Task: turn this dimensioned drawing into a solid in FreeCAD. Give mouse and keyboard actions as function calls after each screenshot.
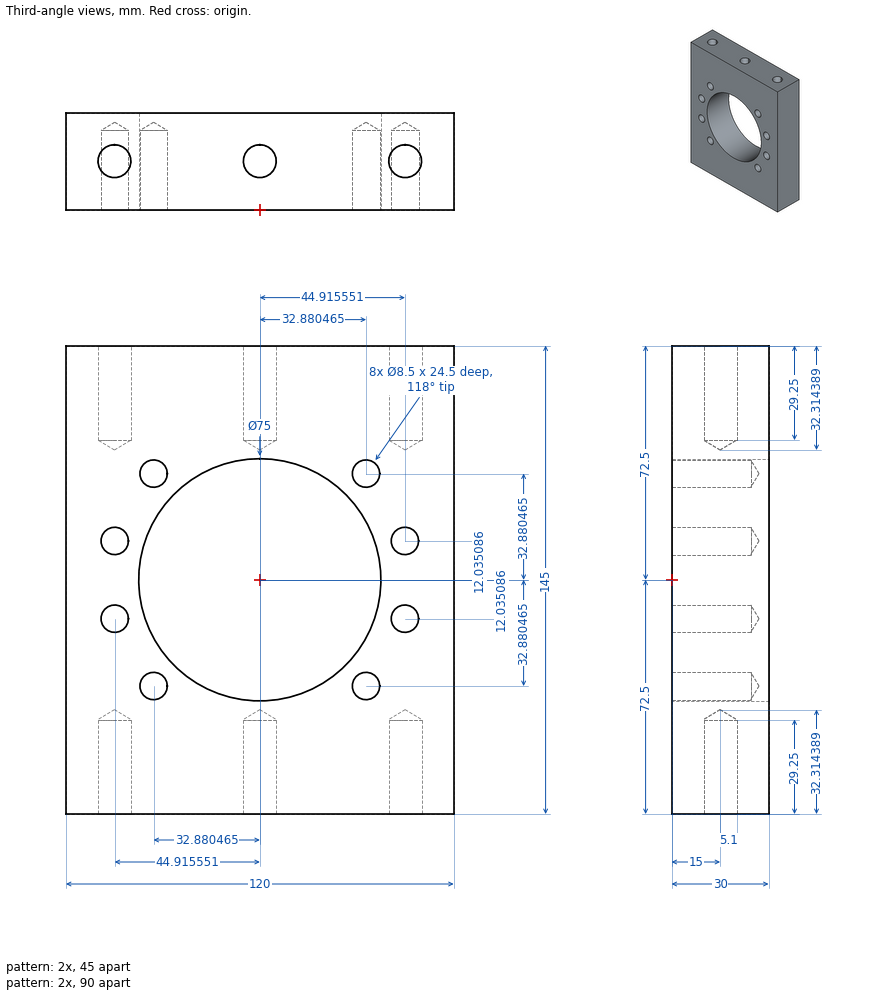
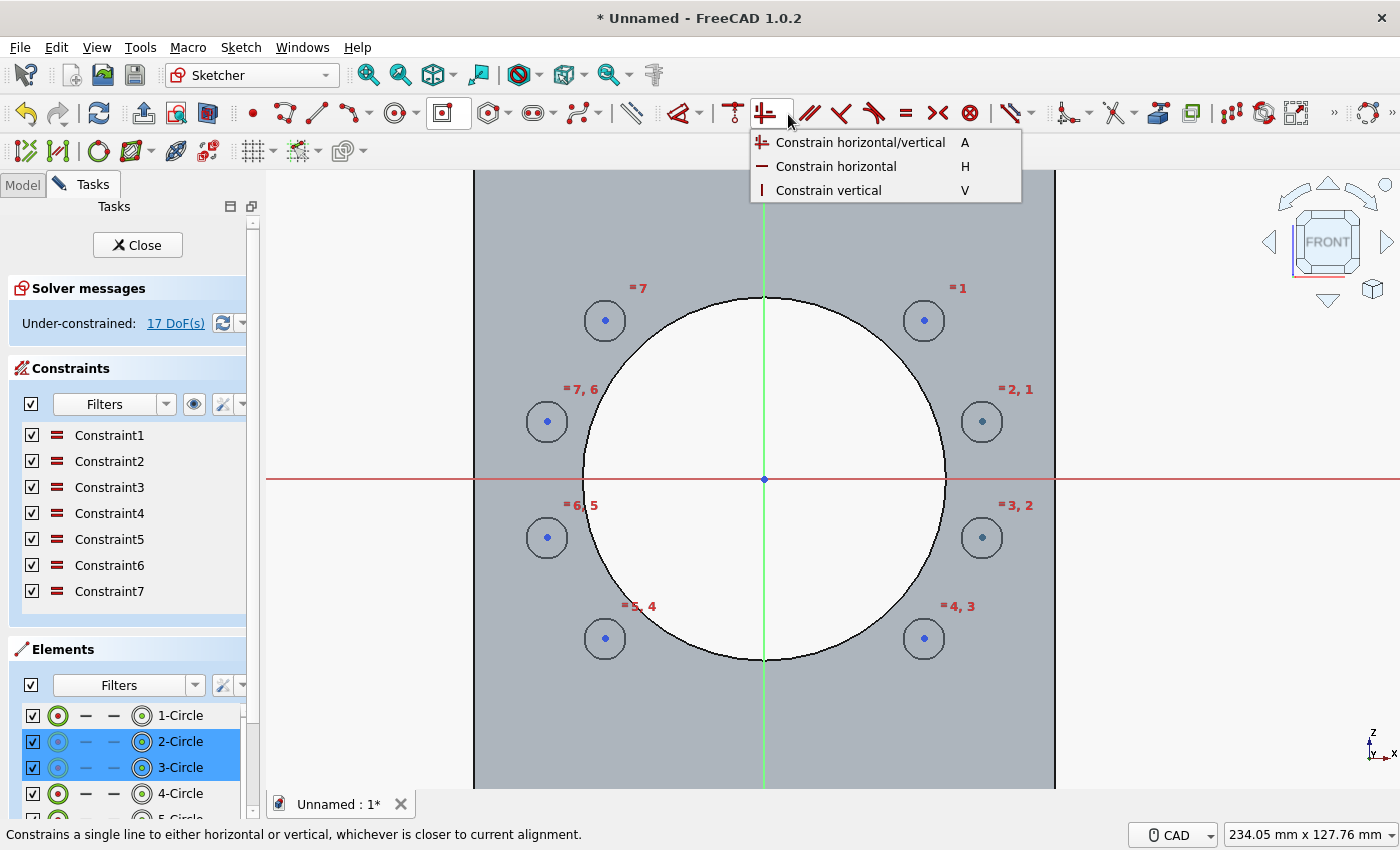
click(886, 190)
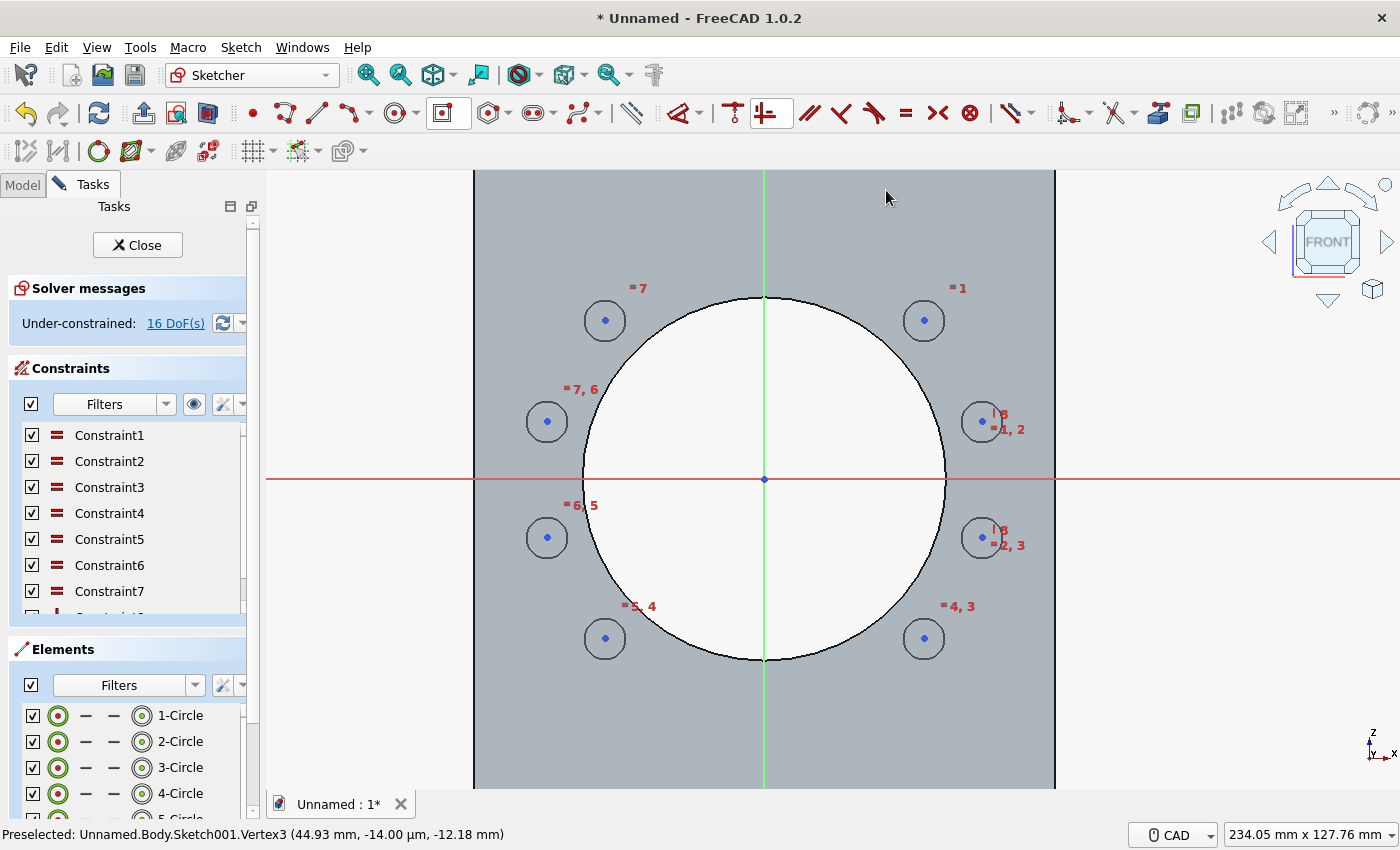
click(924, 321)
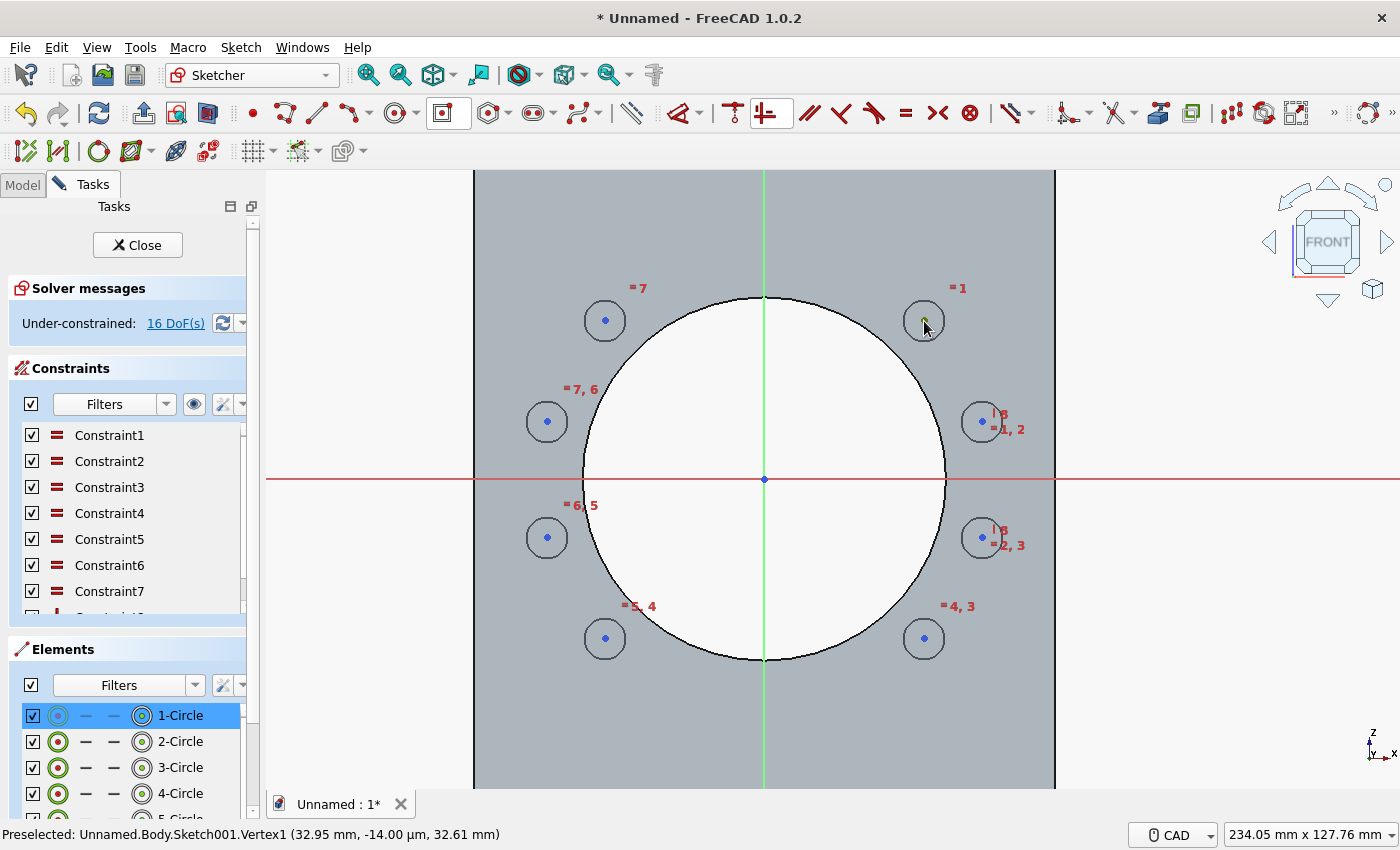
click(924, 639)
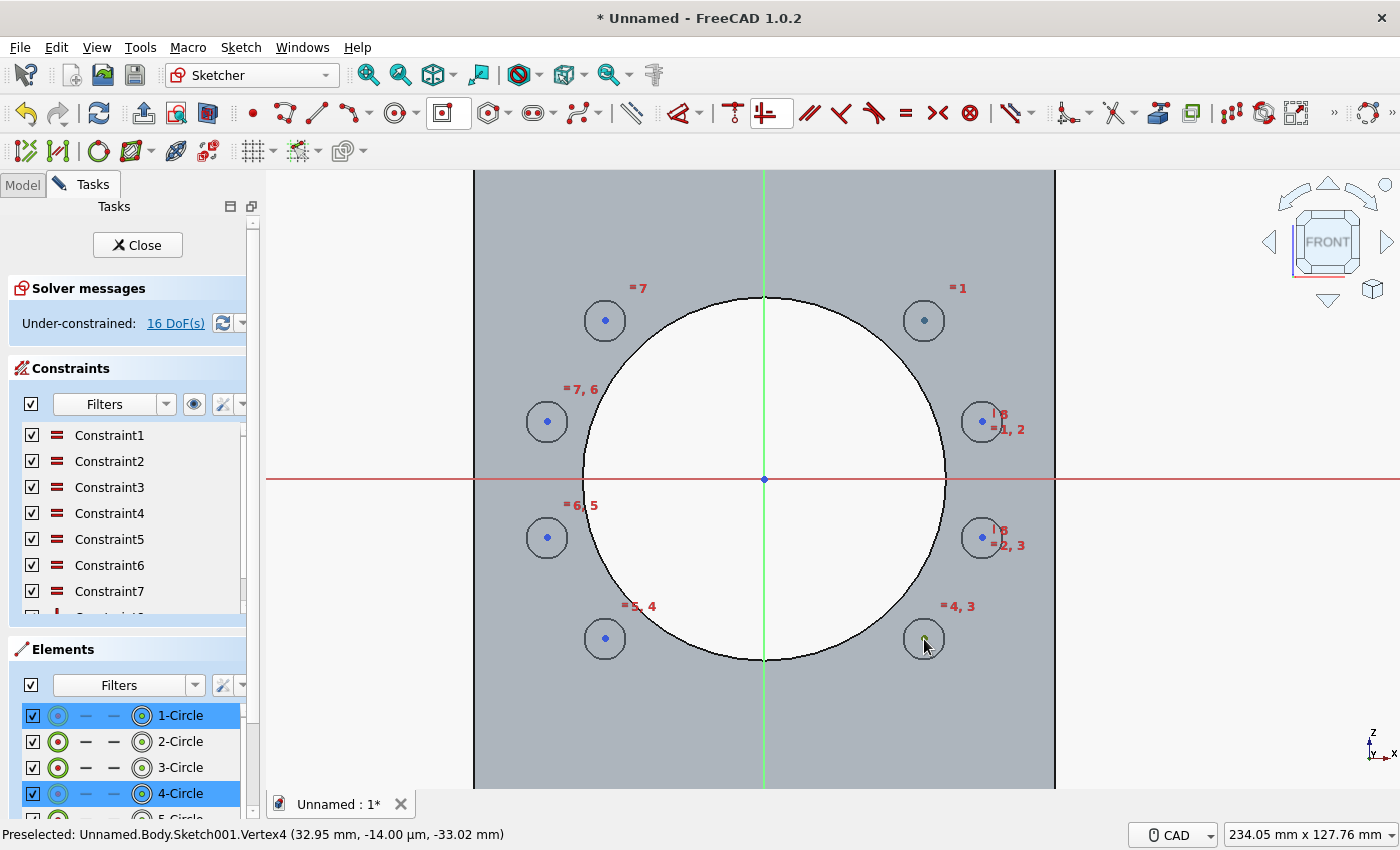
click(788, 114)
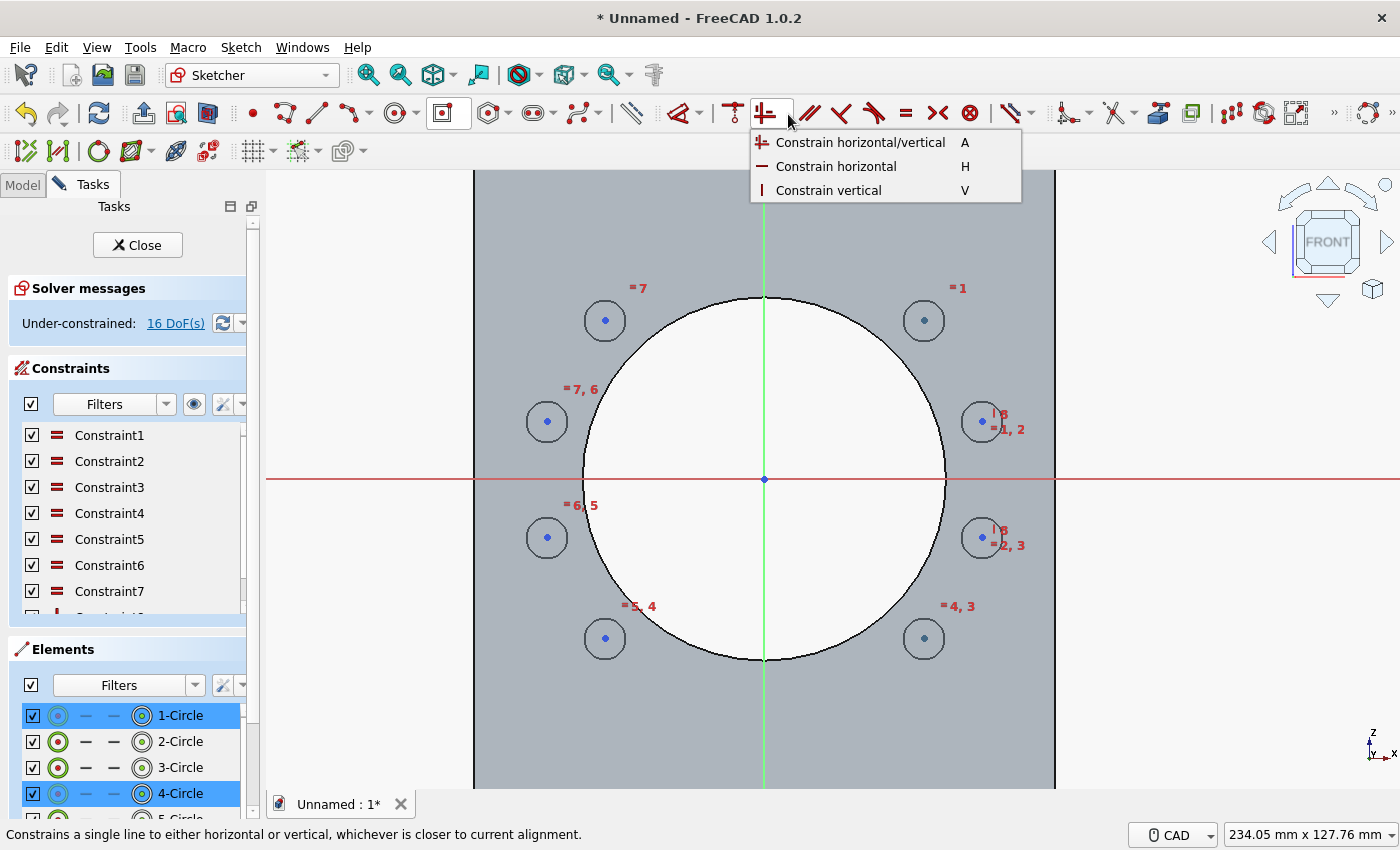
click(886, 190)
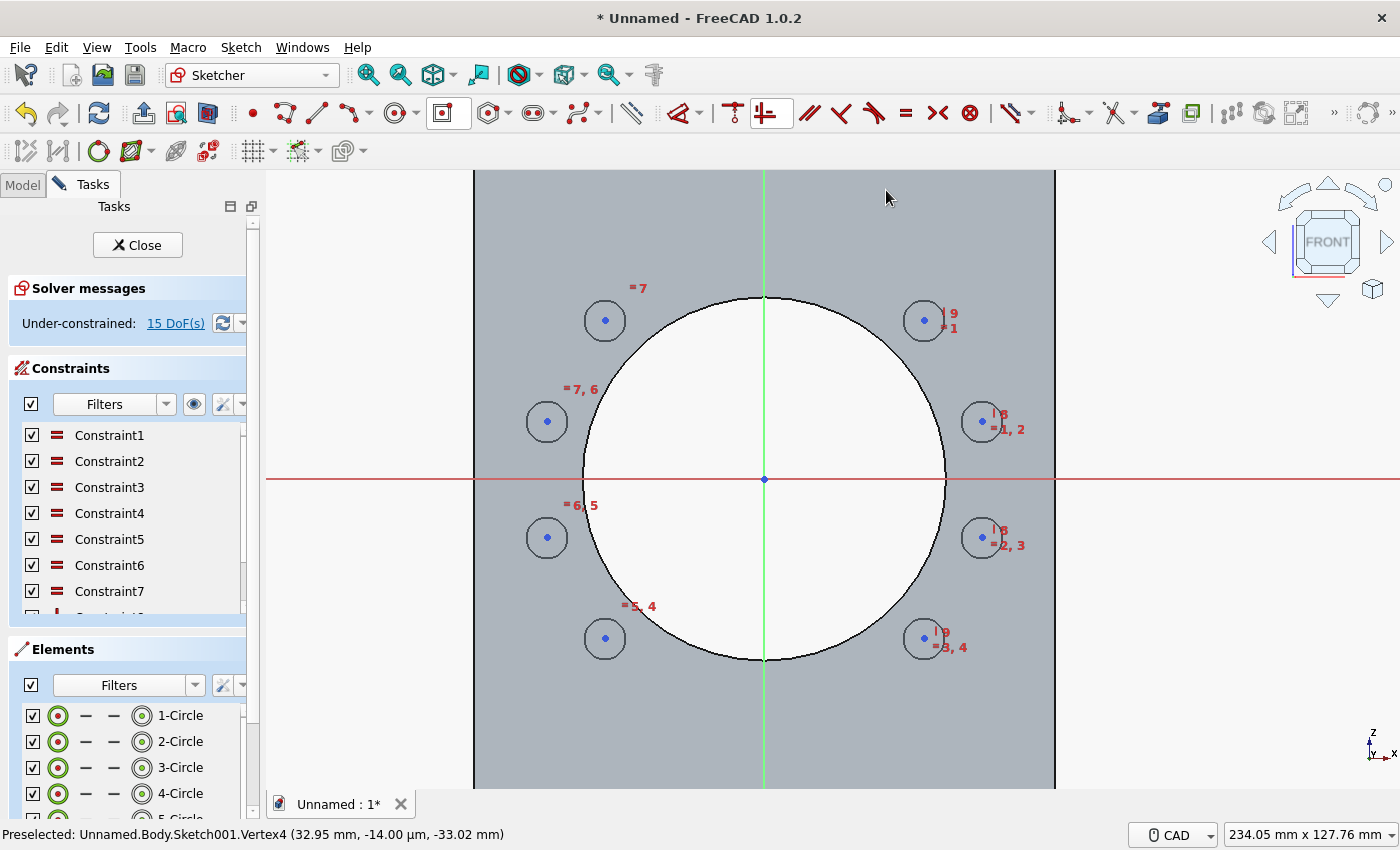
click(924, 639)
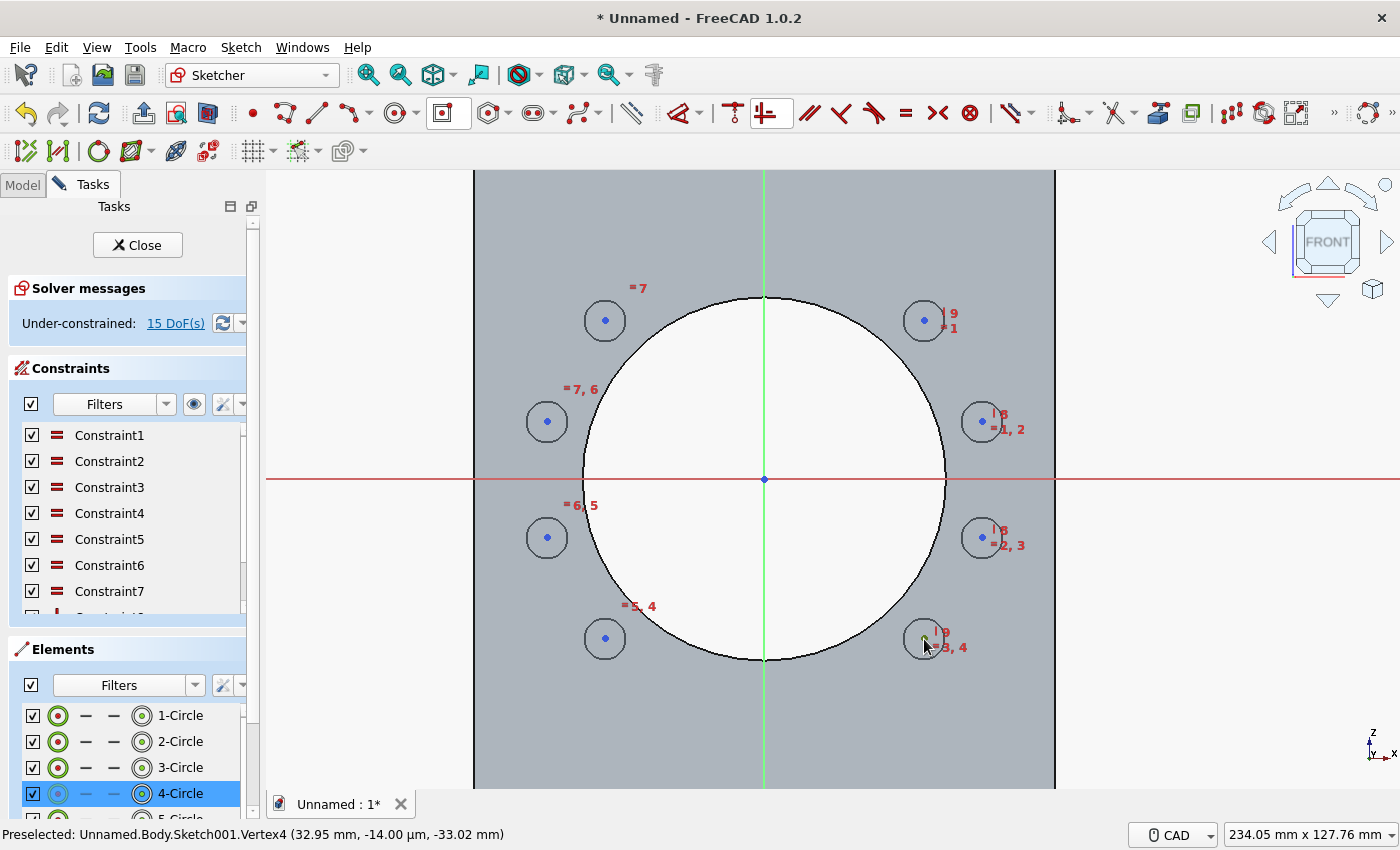
click(605, 639)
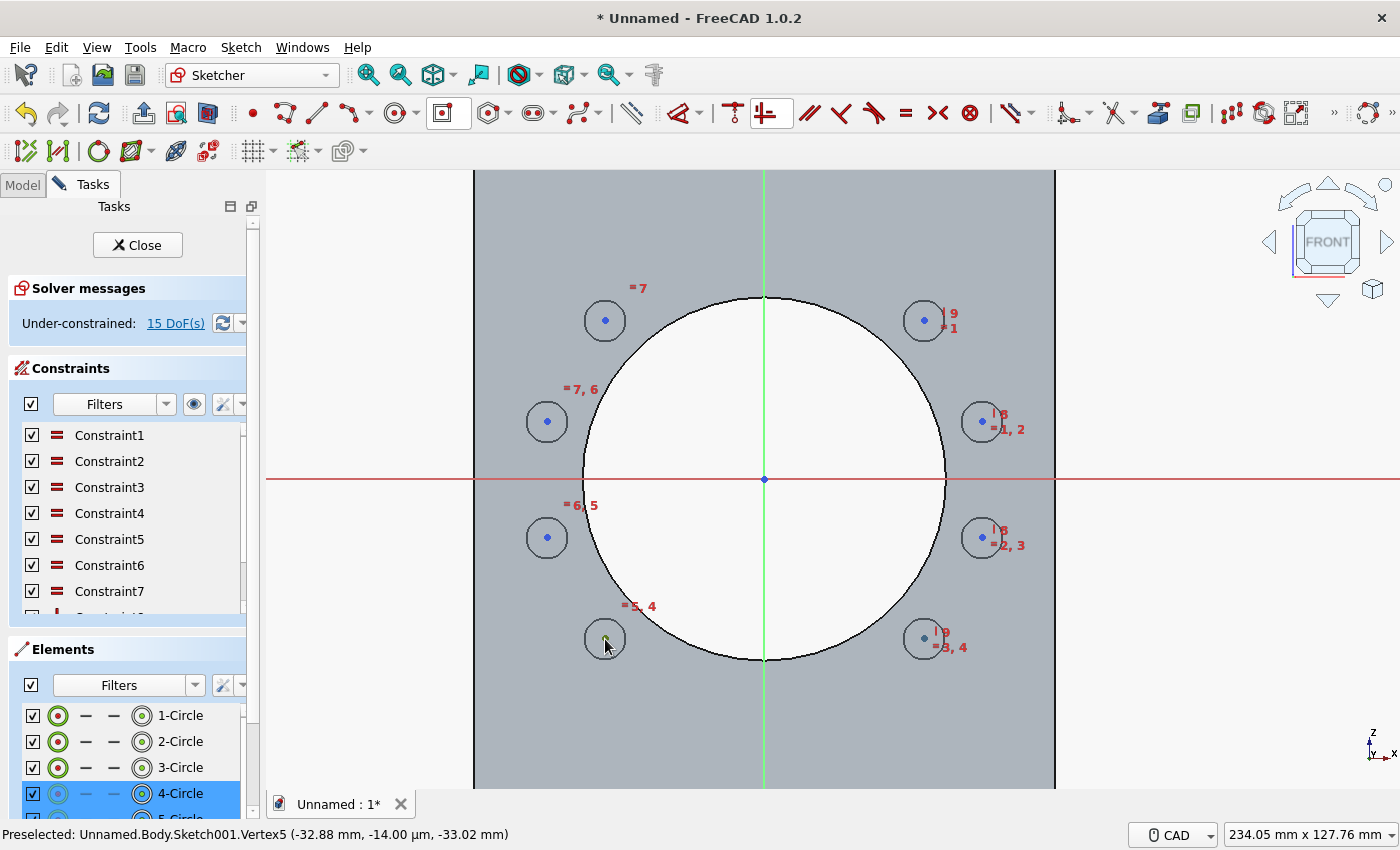
click(788, 114)